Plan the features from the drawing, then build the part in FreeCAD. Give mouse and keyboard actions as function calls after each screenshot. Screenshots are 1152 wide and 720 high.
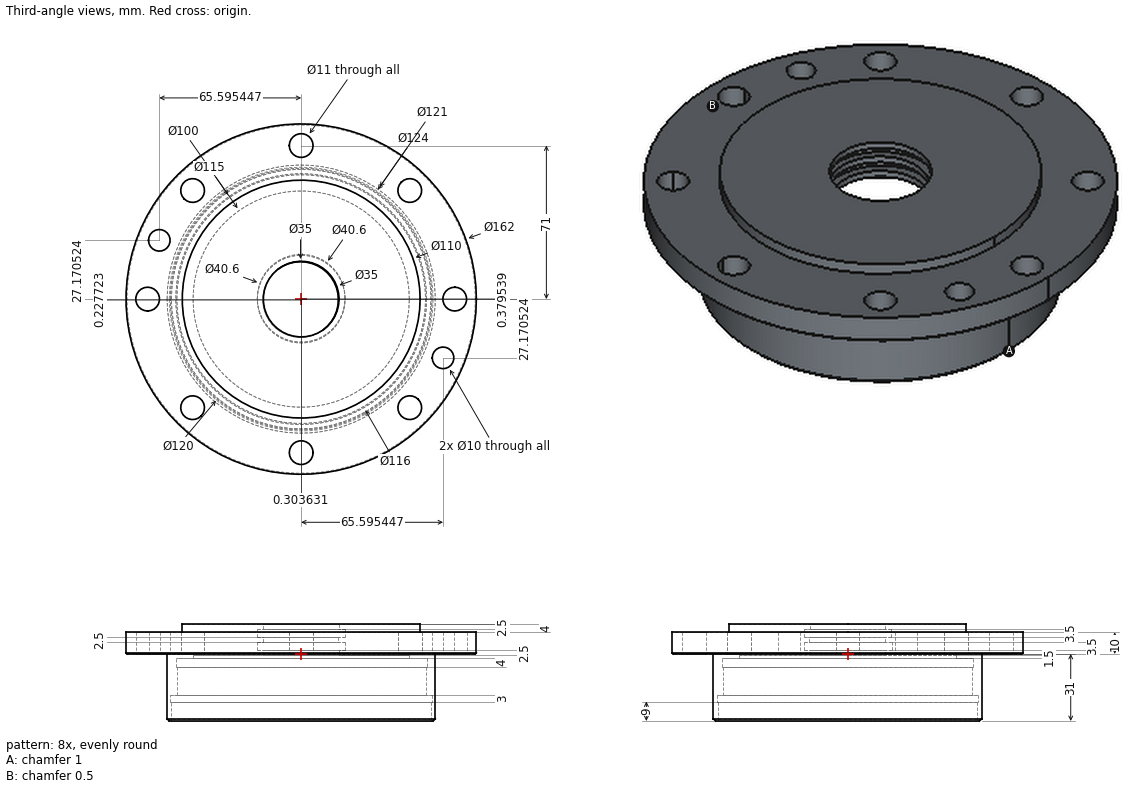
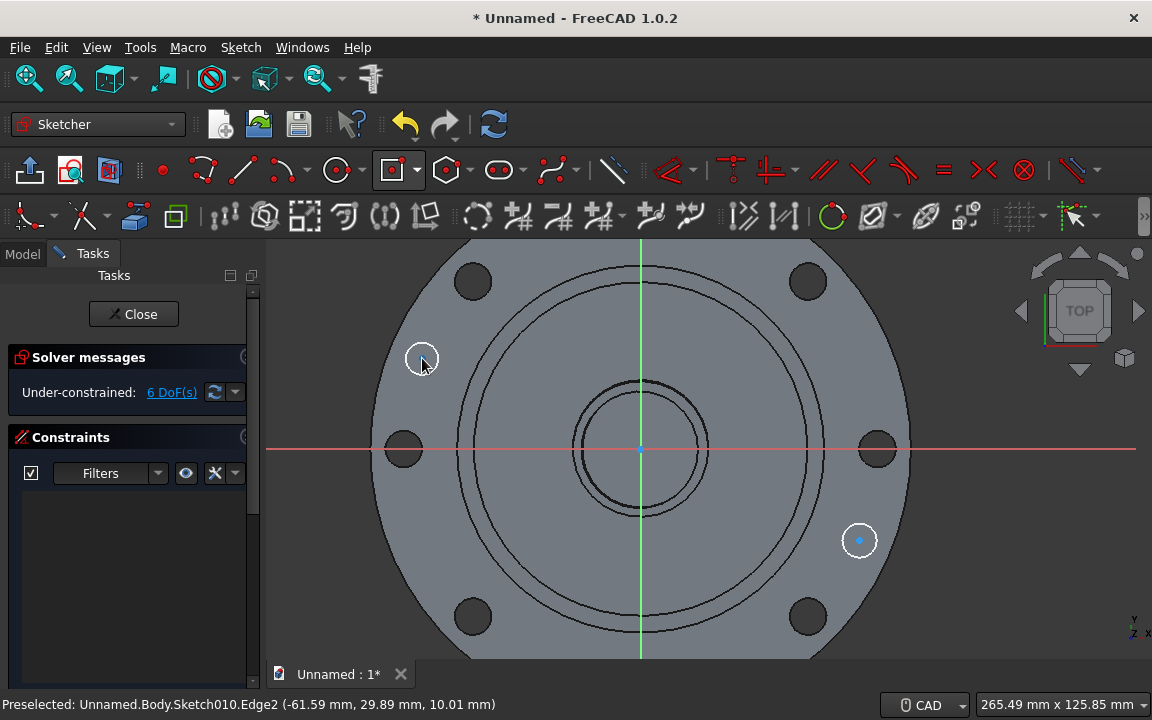
click(872, 528)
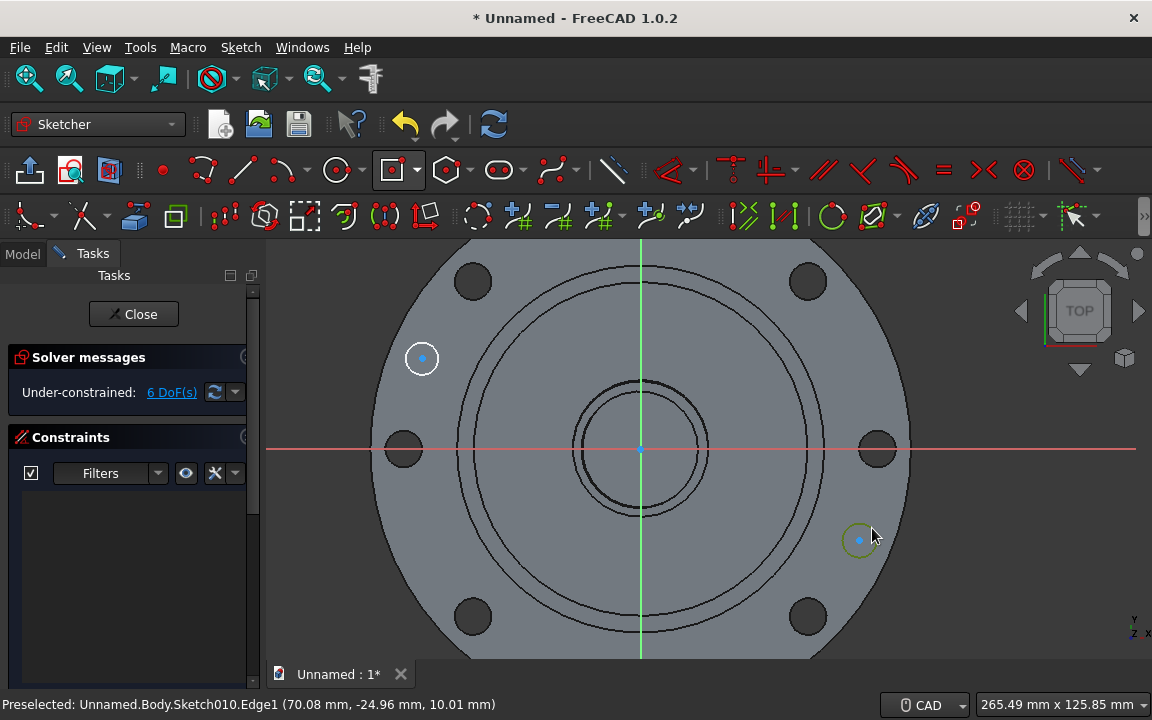
click(433, 347)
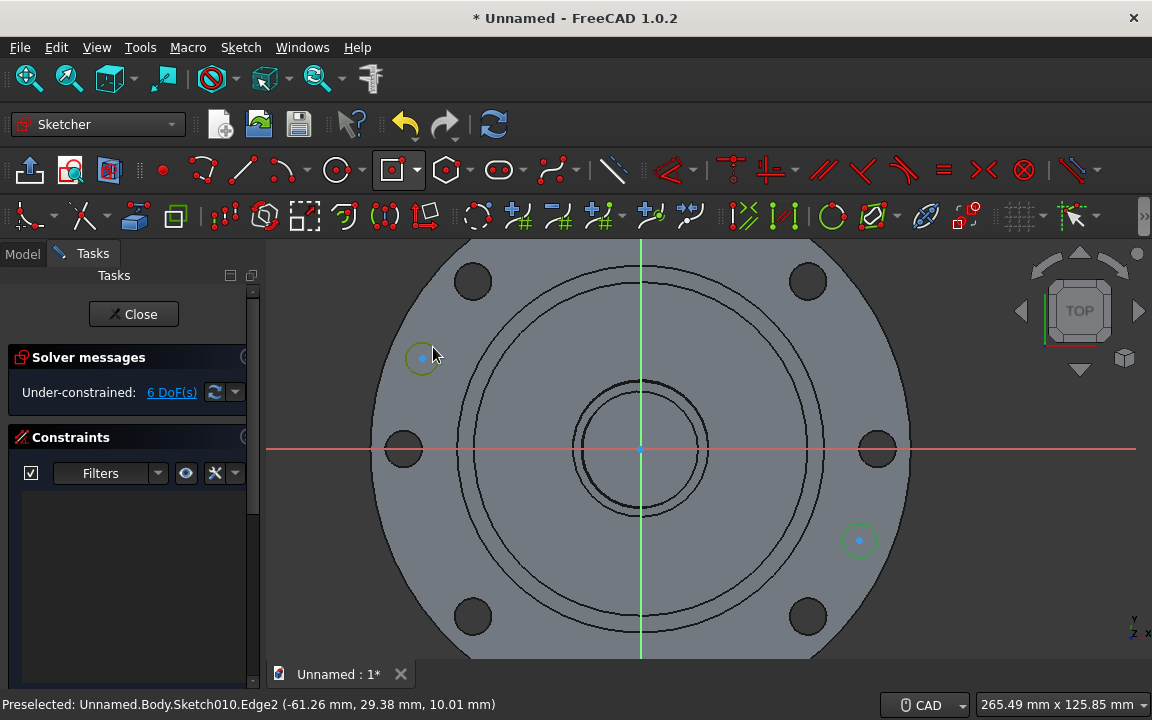
click(944, 170)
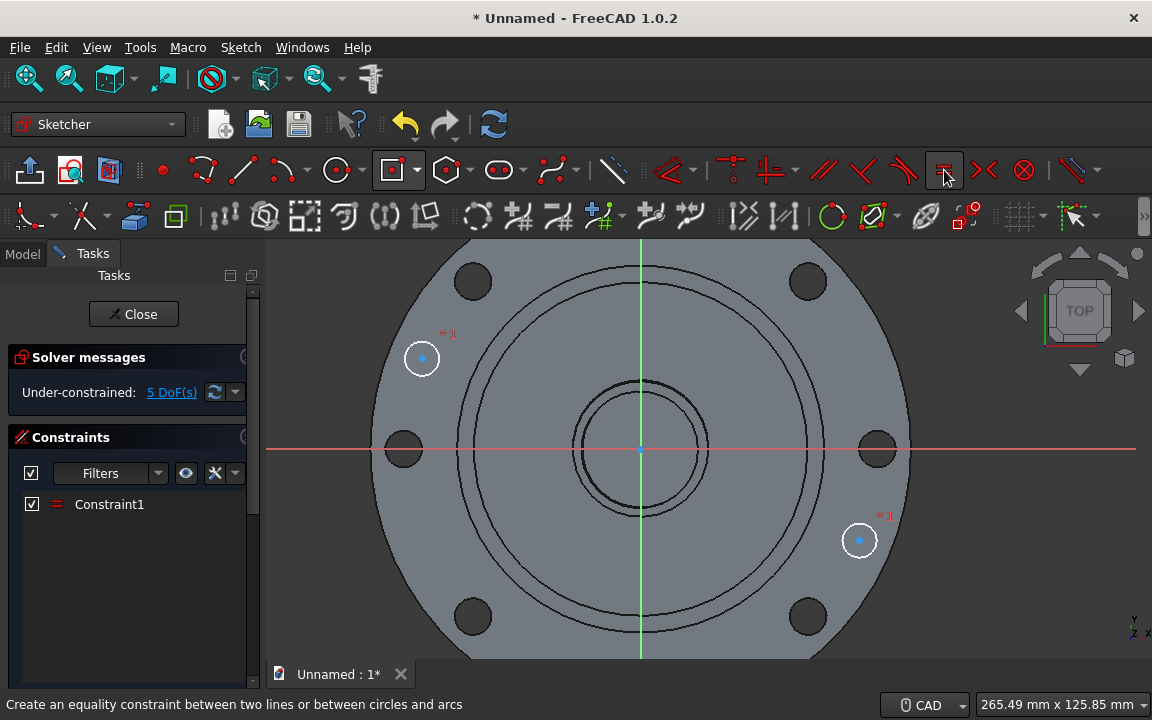
key(d)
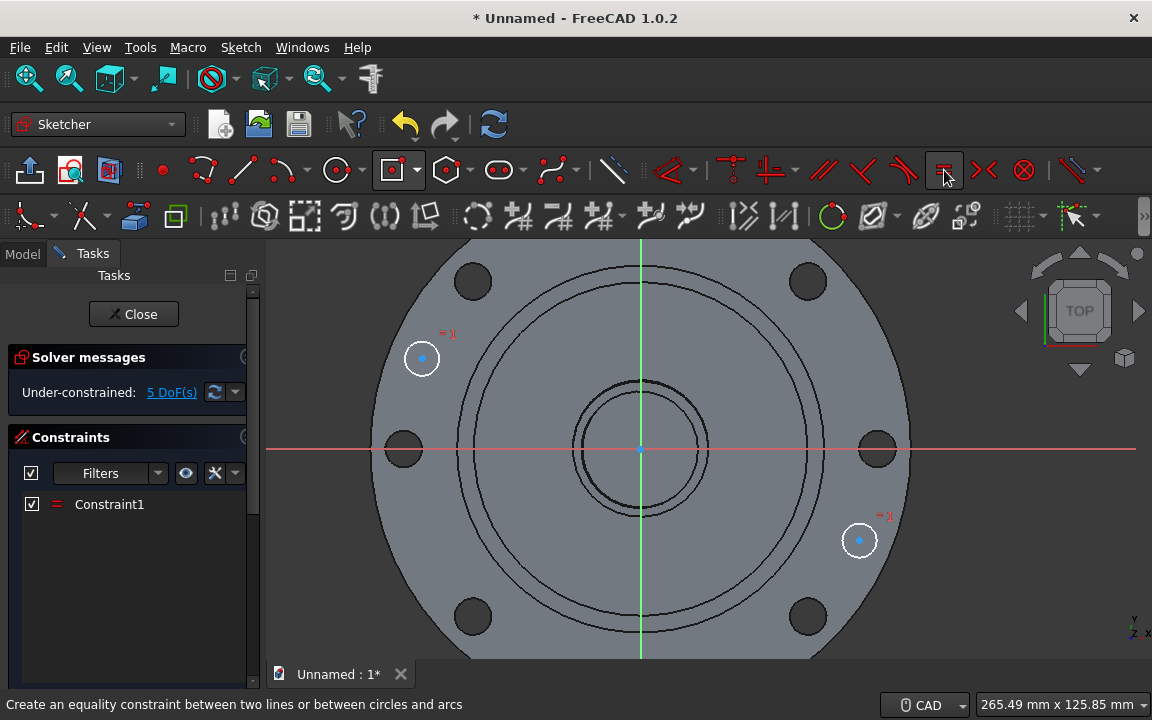
click(872, 528)
click(895, 505)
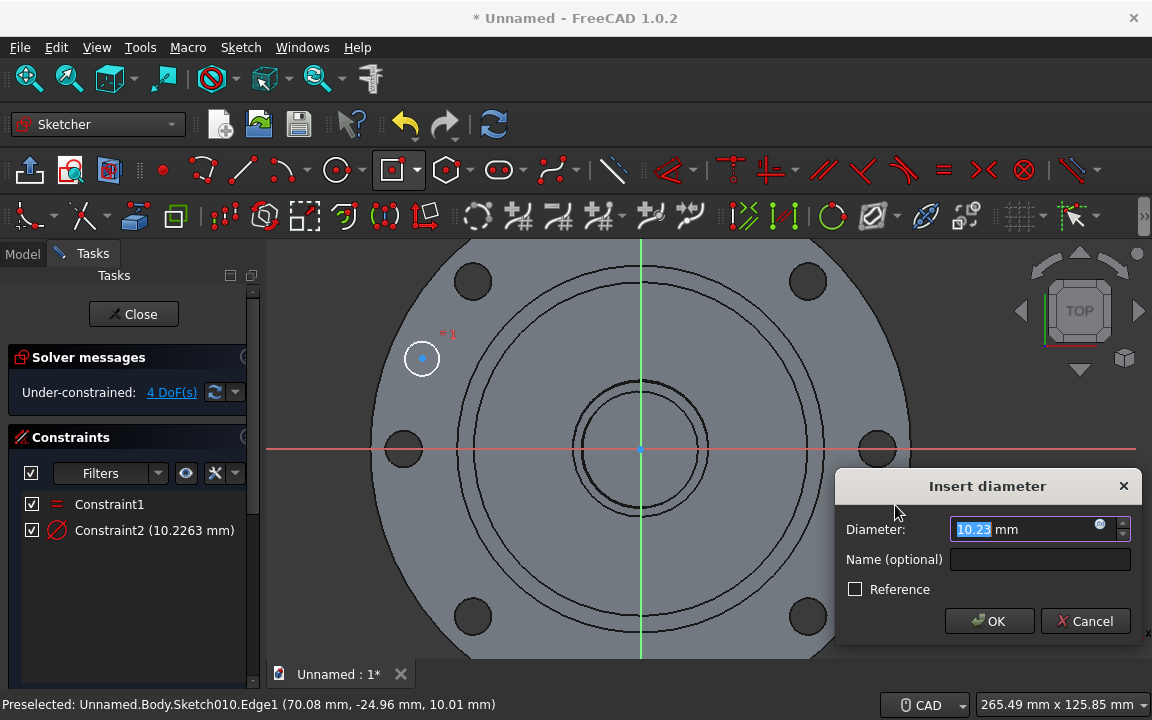
text(10)
key(Return)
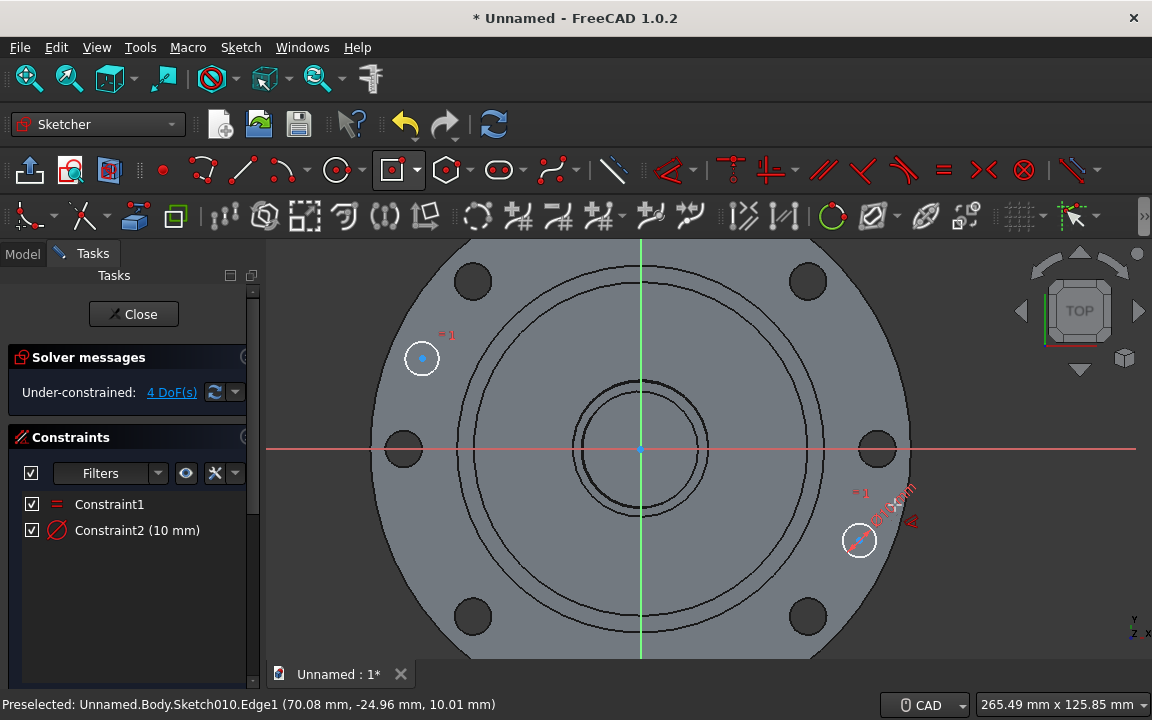
click(860, 541)
click(750, 575)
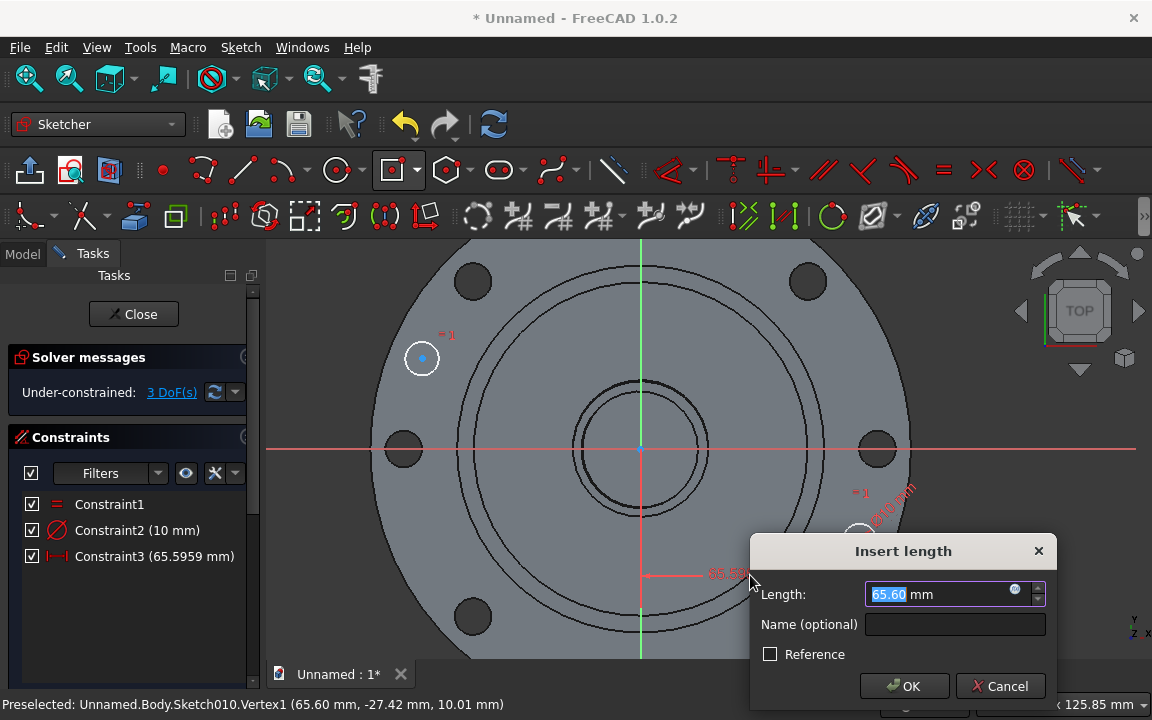
text(65.595447)
key(Return)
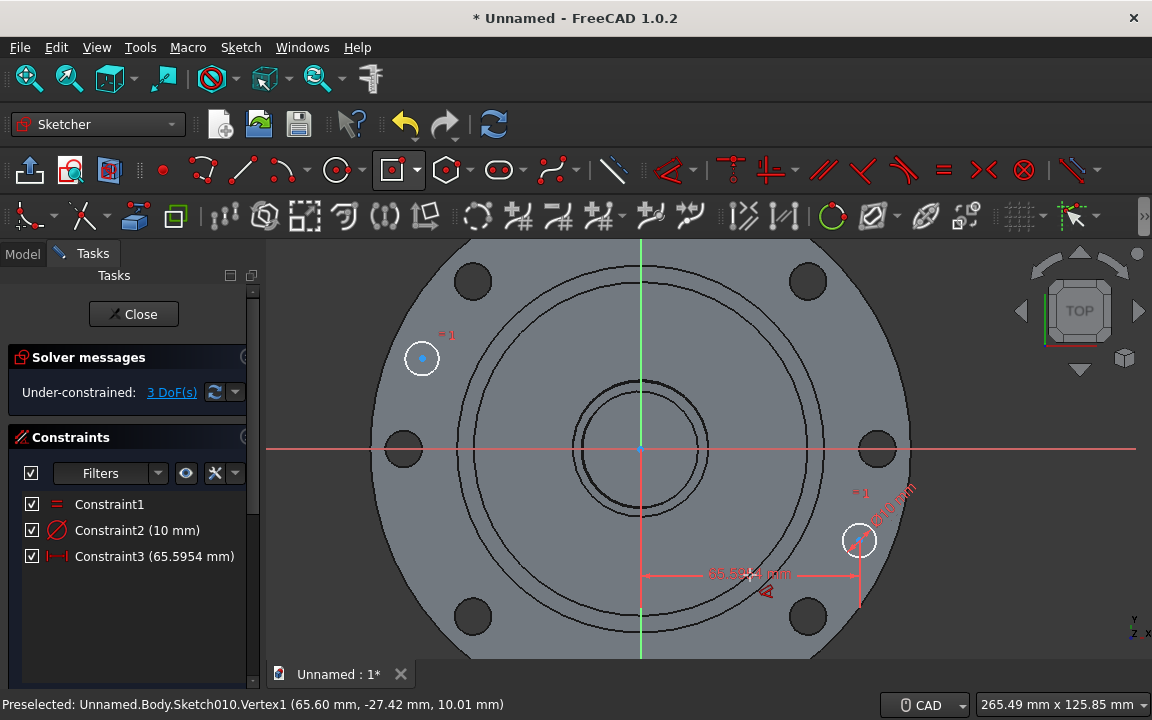
click(860, 541)
click(894, 474)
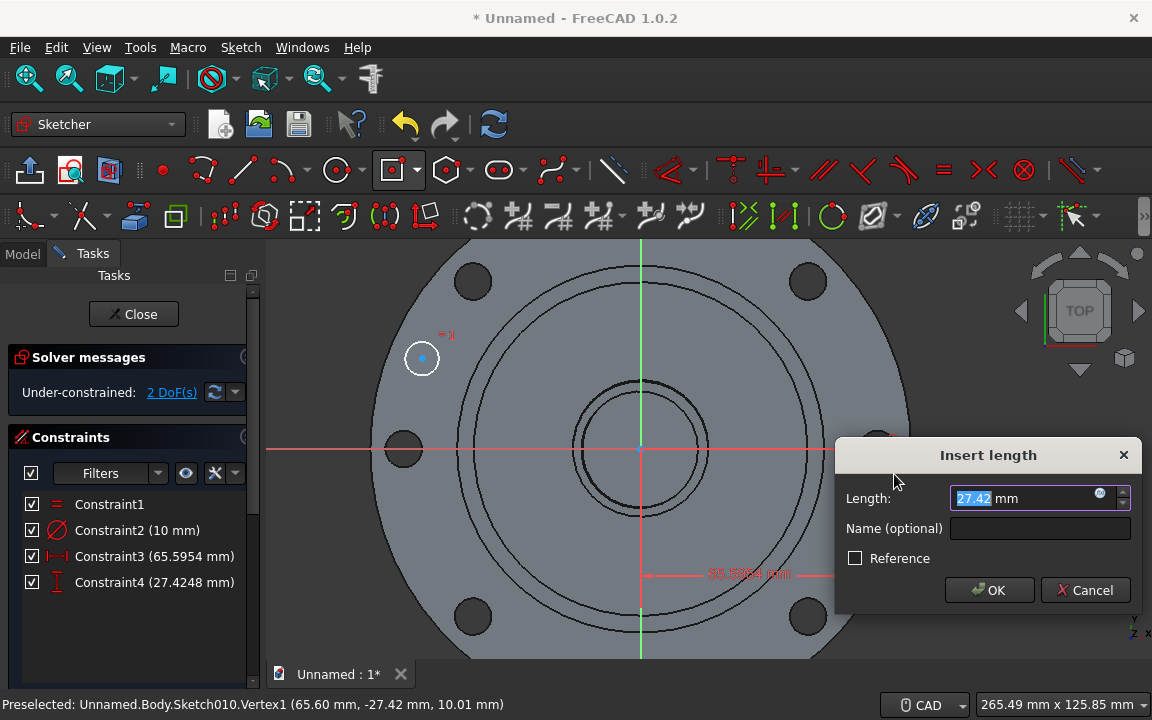
text(27.170524)
key(Return)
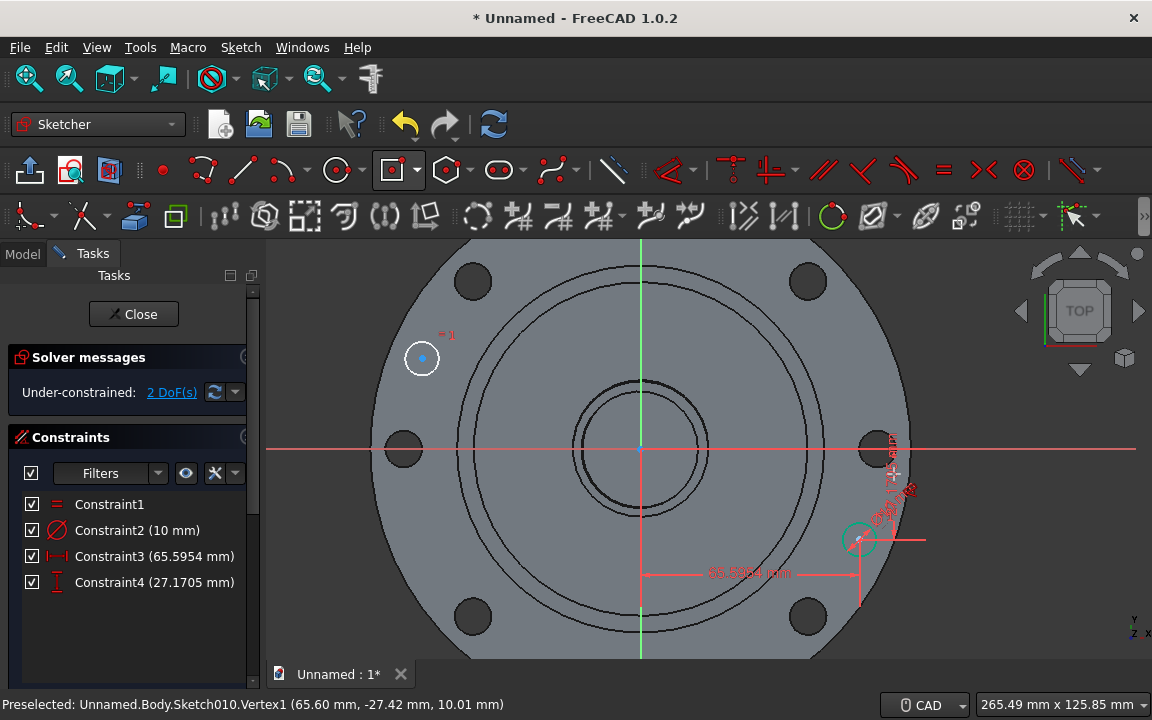
click(422, 359)
click(531, 325)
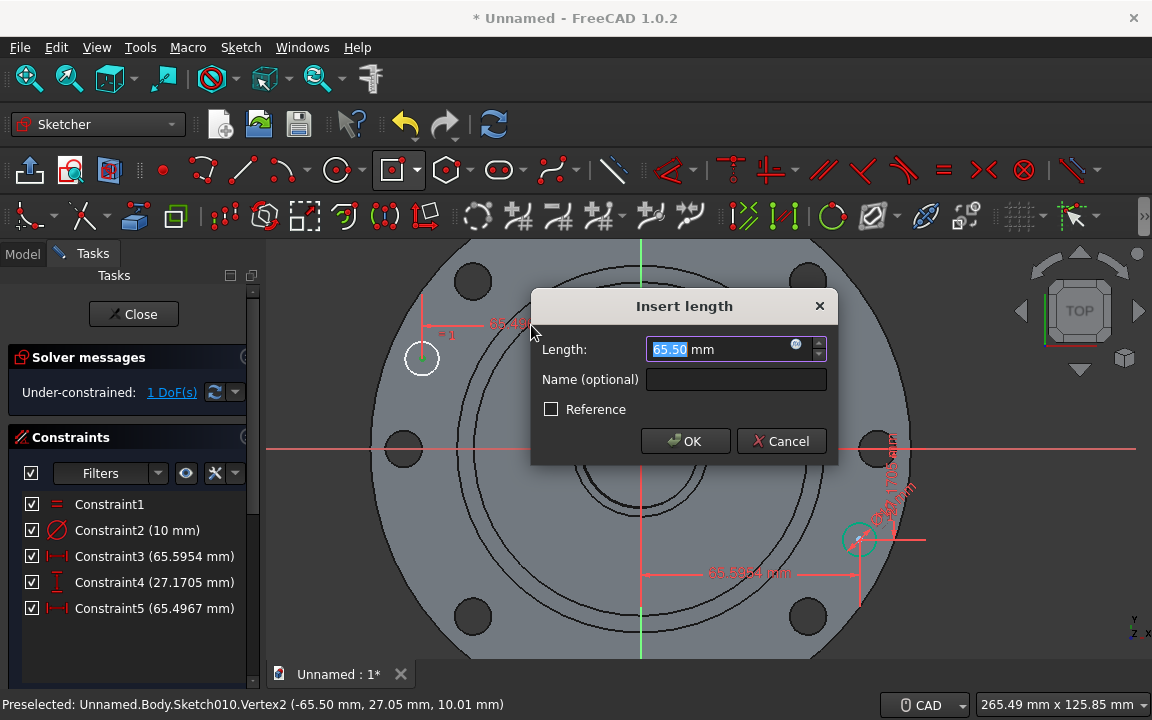
text(65.595447)
key(Return)